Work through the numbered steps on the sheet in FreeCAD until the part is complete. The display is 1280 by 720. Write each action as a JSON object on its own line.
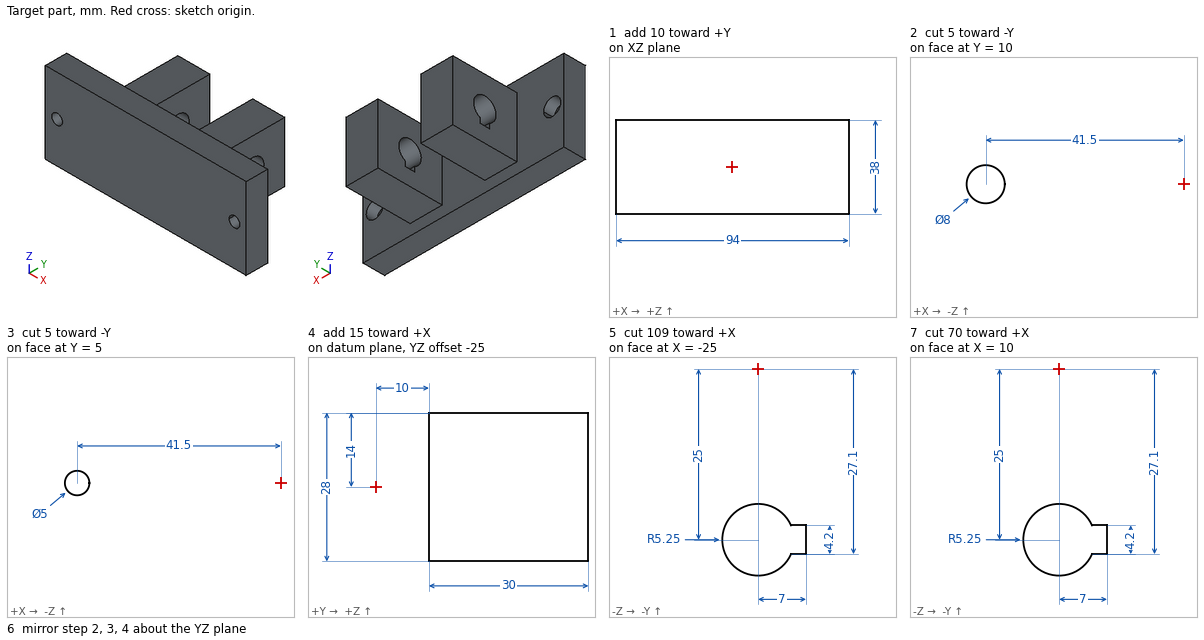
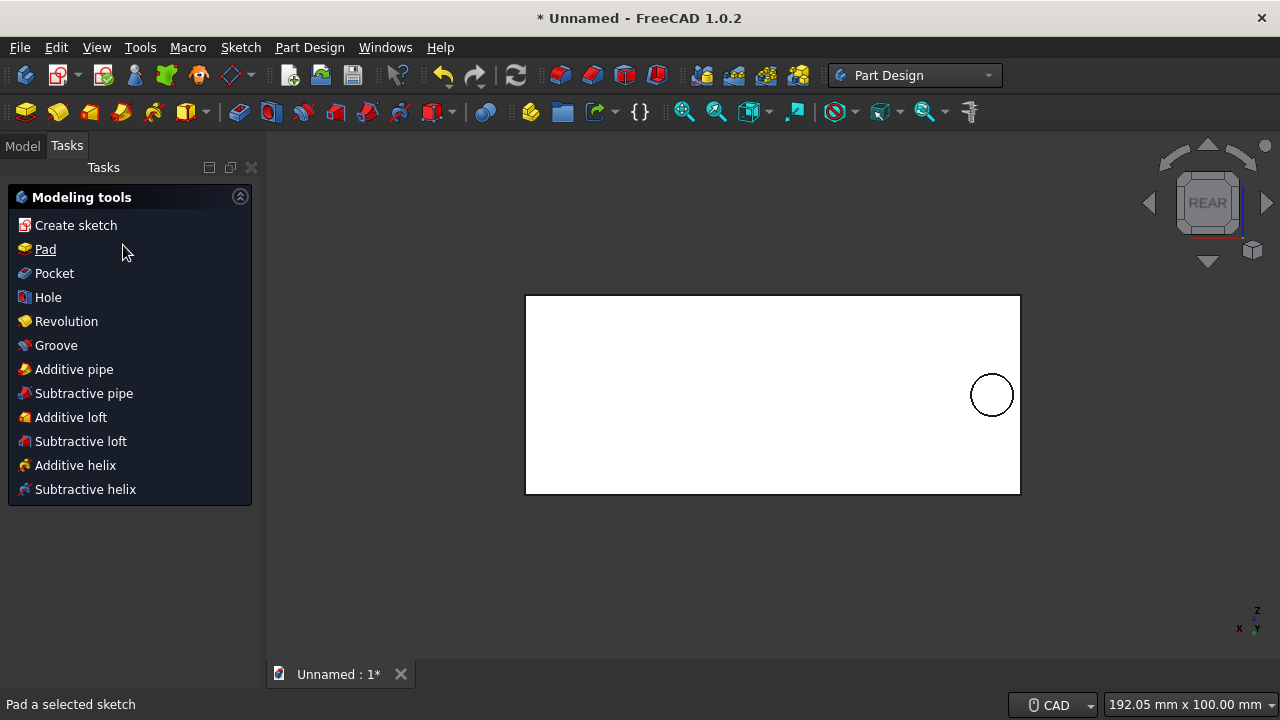
{"action": "left_click", "coordinate": [240, 112]}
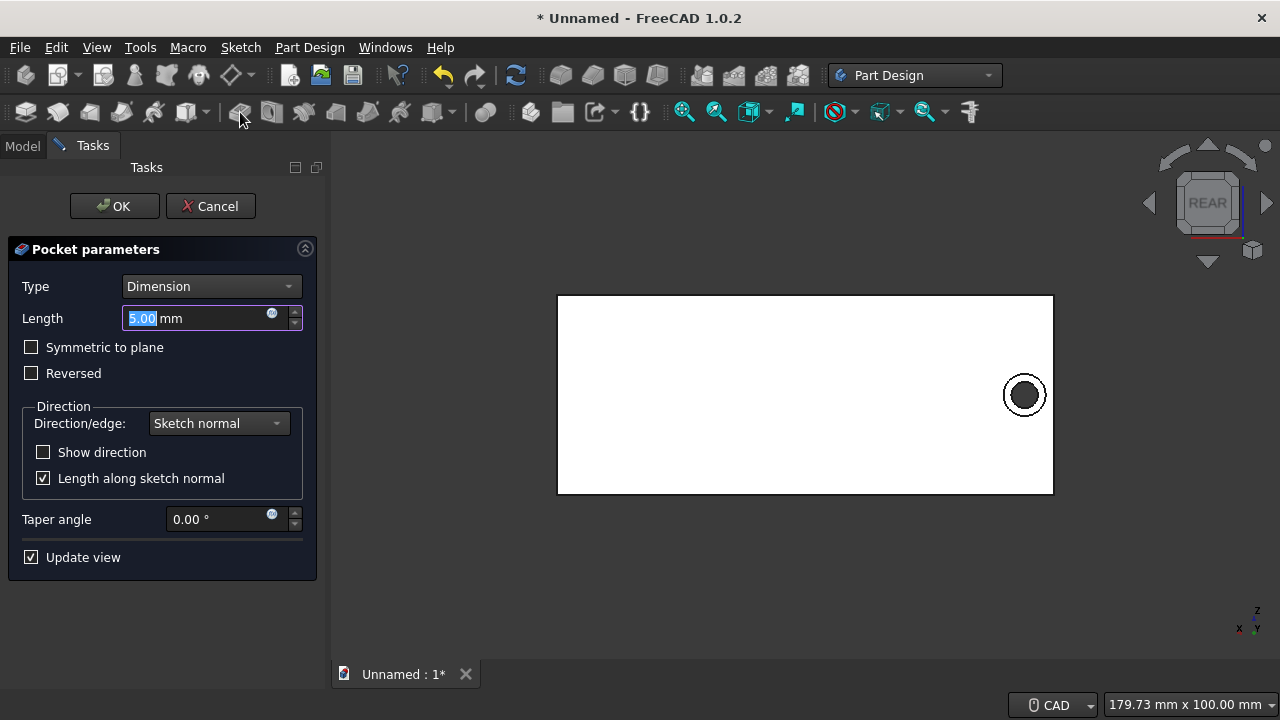
{"action": "type", "text": "5"}
{"action": "key", "text": "Tab"}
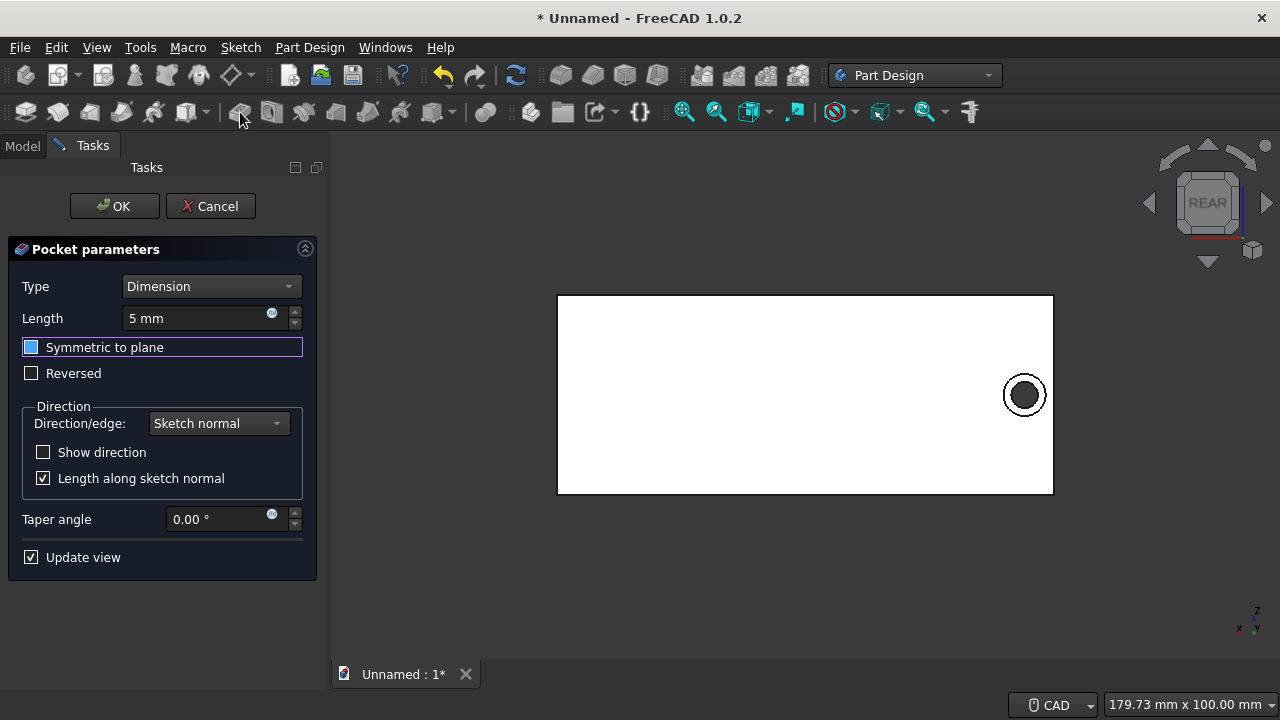
{"action": "left_click", "coordinate": [115, 206]}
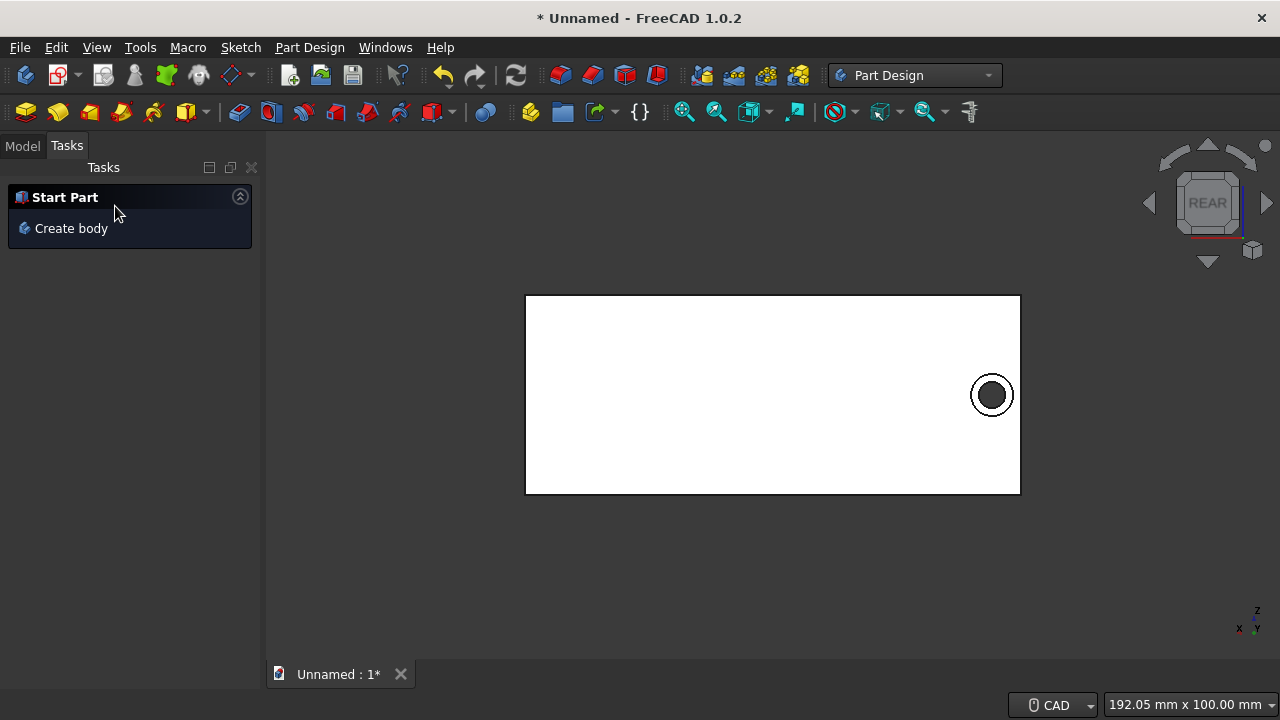
{"action": "left_click", "coordinate": [23, 145]}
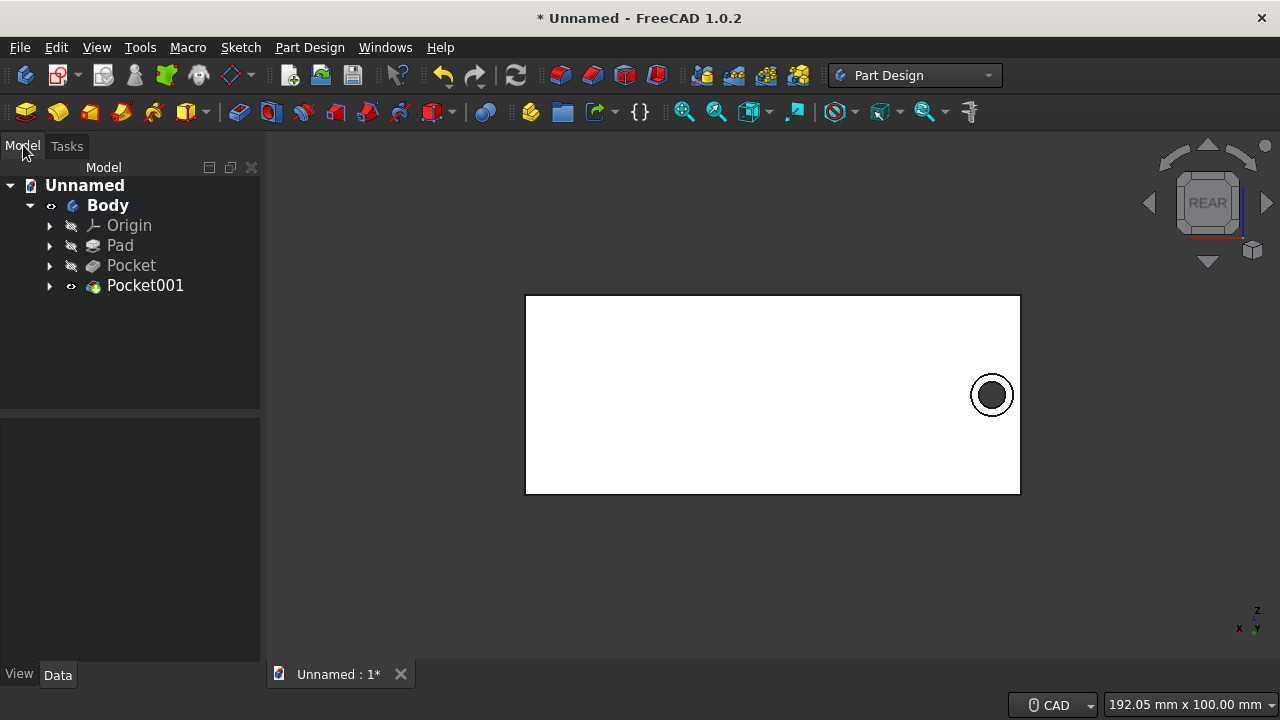
{"action": "left_click", "coordinate": [50, 226]}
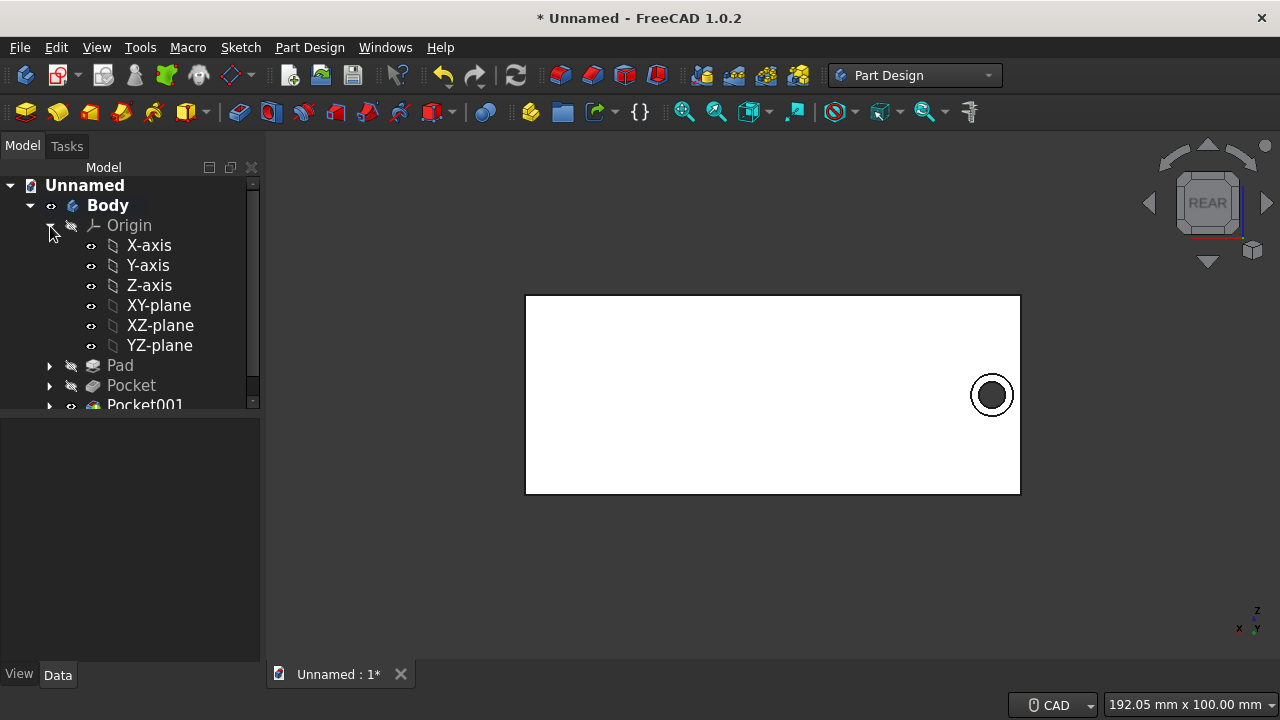
{"action": "left_click", "coordinate": [136, 346]}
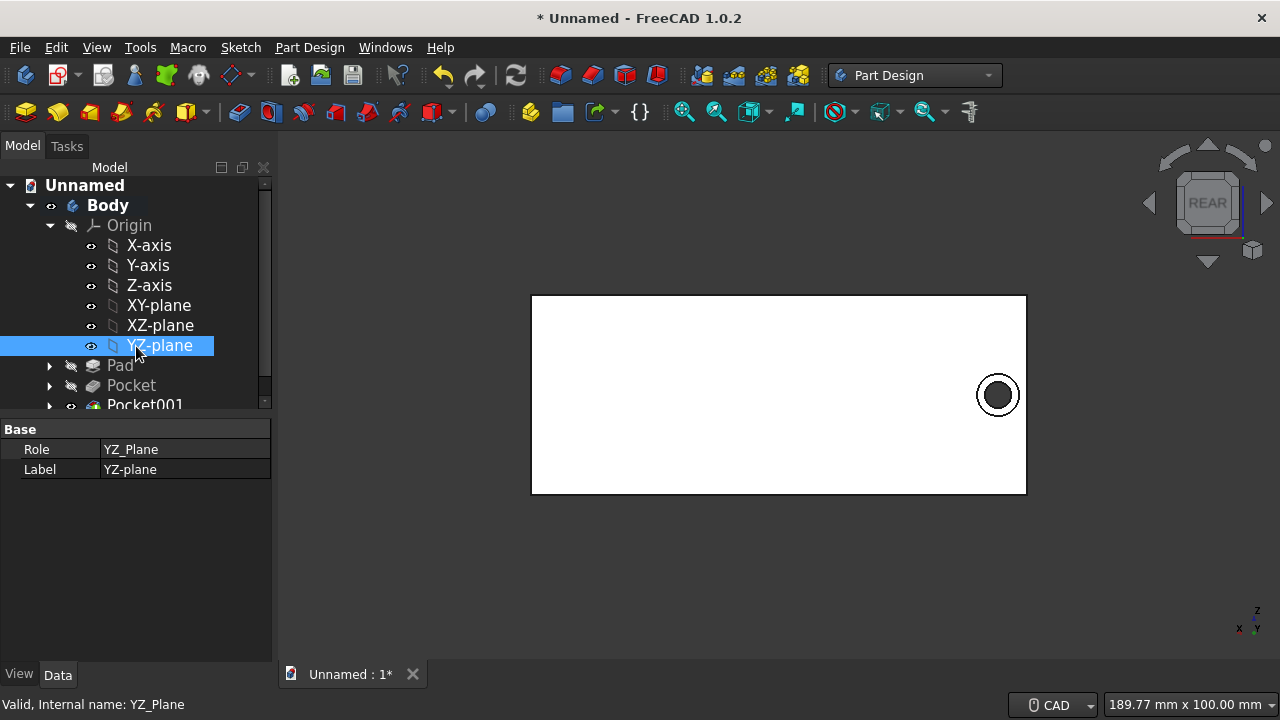
{"action": "left_click", "coordinate": [232, 76]}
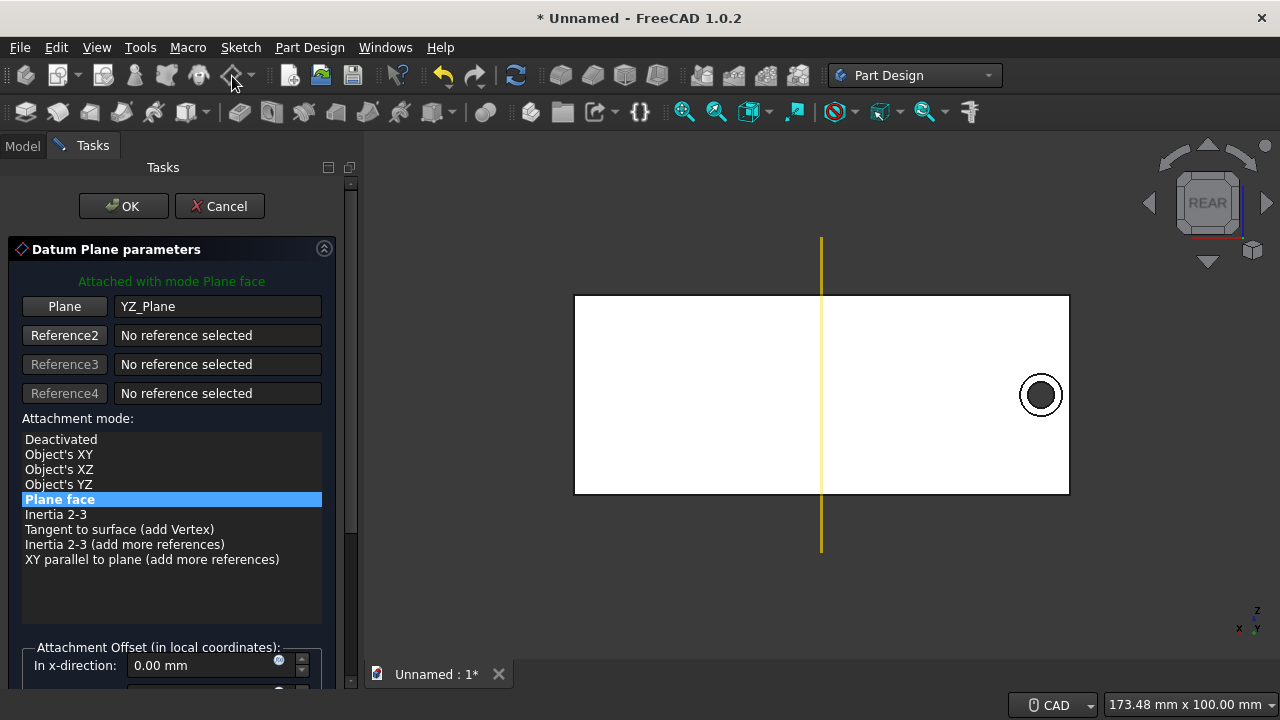
{"action": "scroll", "coordinate": [351, 432], "scroll_direction": "down", "scroll_amount": 2}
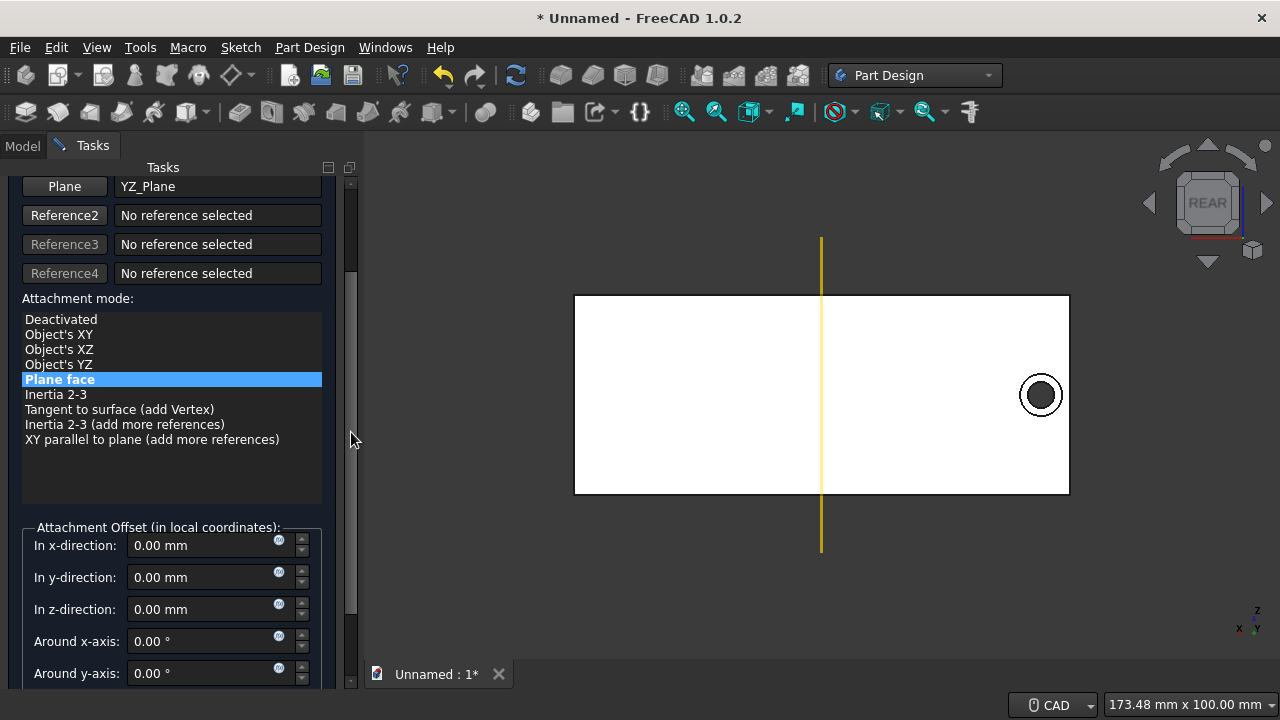
{"action": "triple_click", "coordinate": [210, 609]}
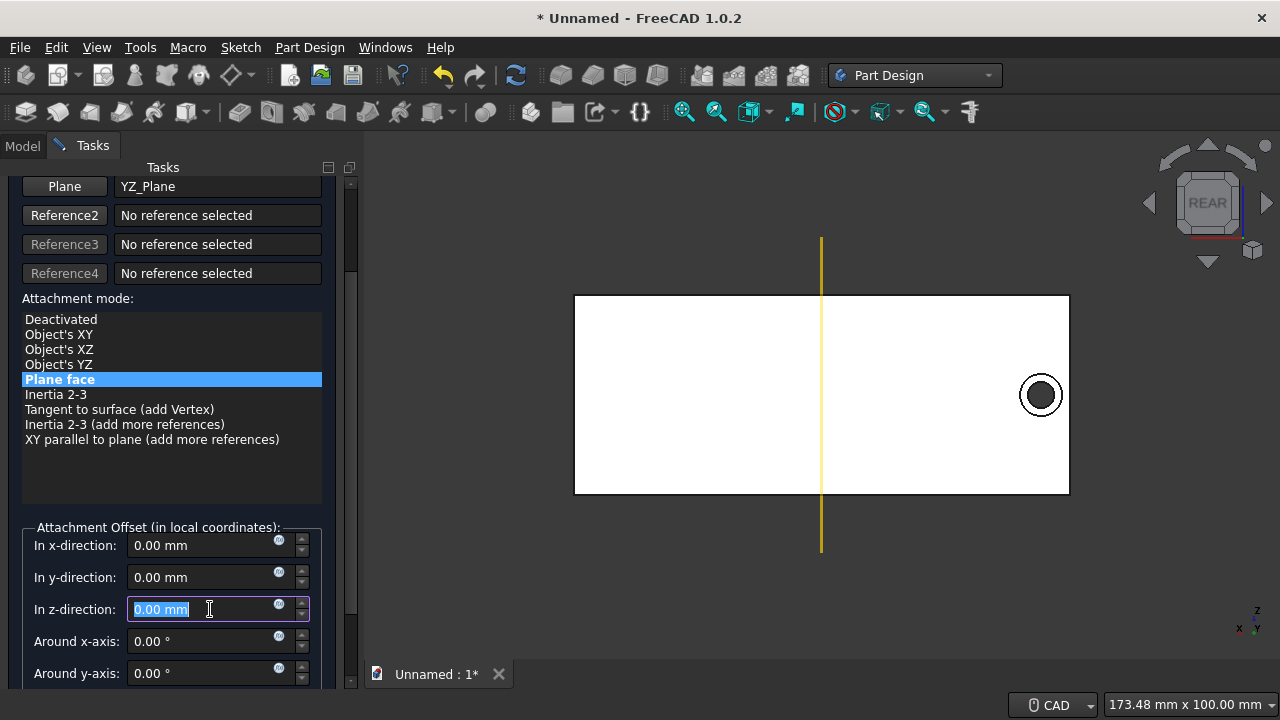
{"action": "type", "text": "-25"}
{"action": "key", "text": "Tab"}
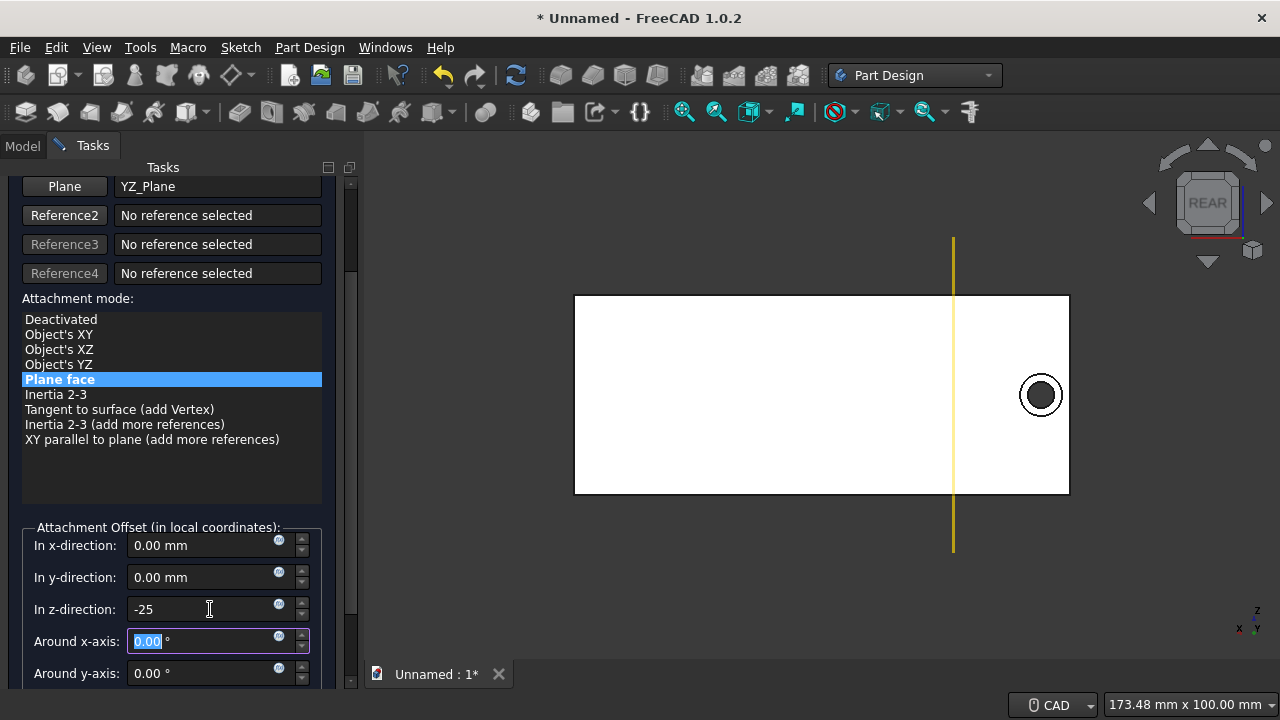
{"action": "scroll", "coordinate": [351, 432], "scroll_direction": "up", "scroll_amount": 3}